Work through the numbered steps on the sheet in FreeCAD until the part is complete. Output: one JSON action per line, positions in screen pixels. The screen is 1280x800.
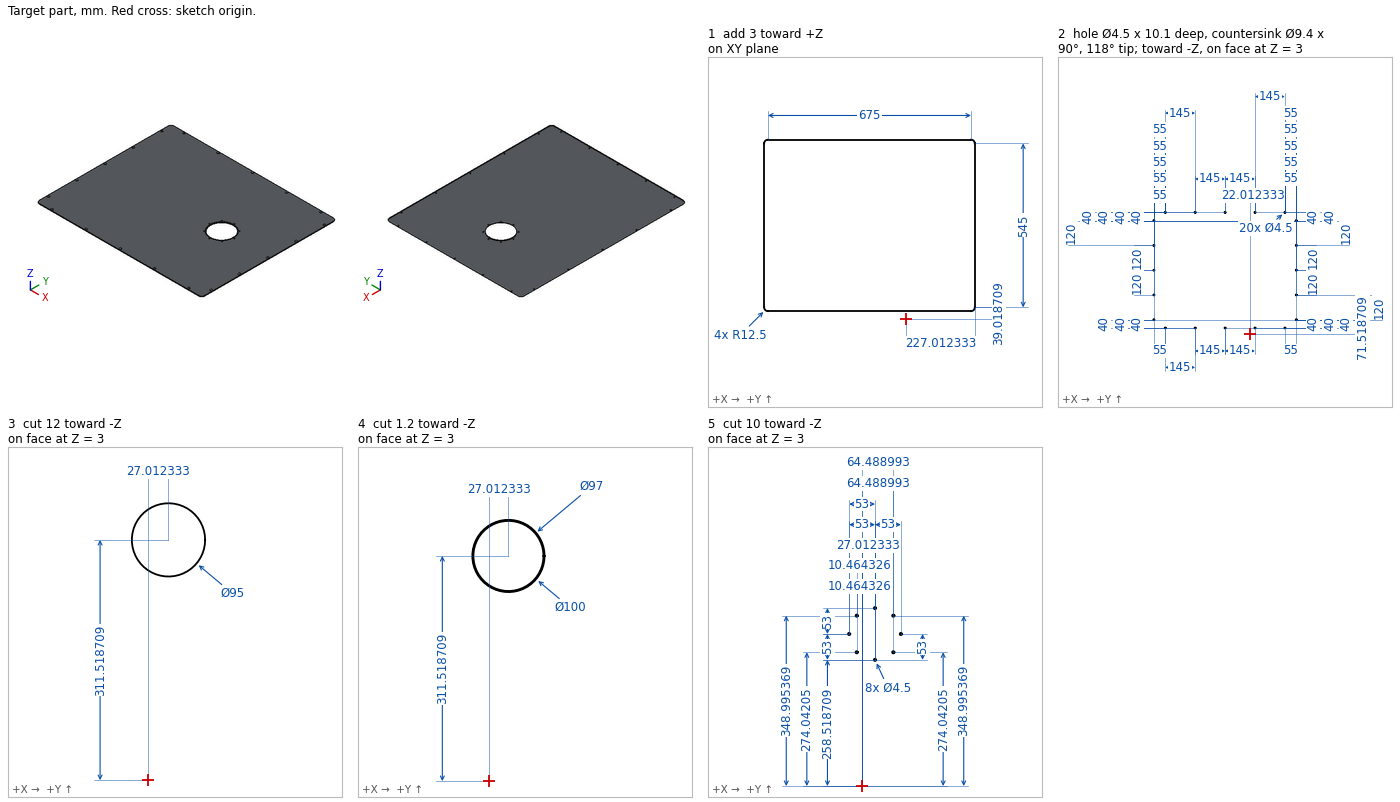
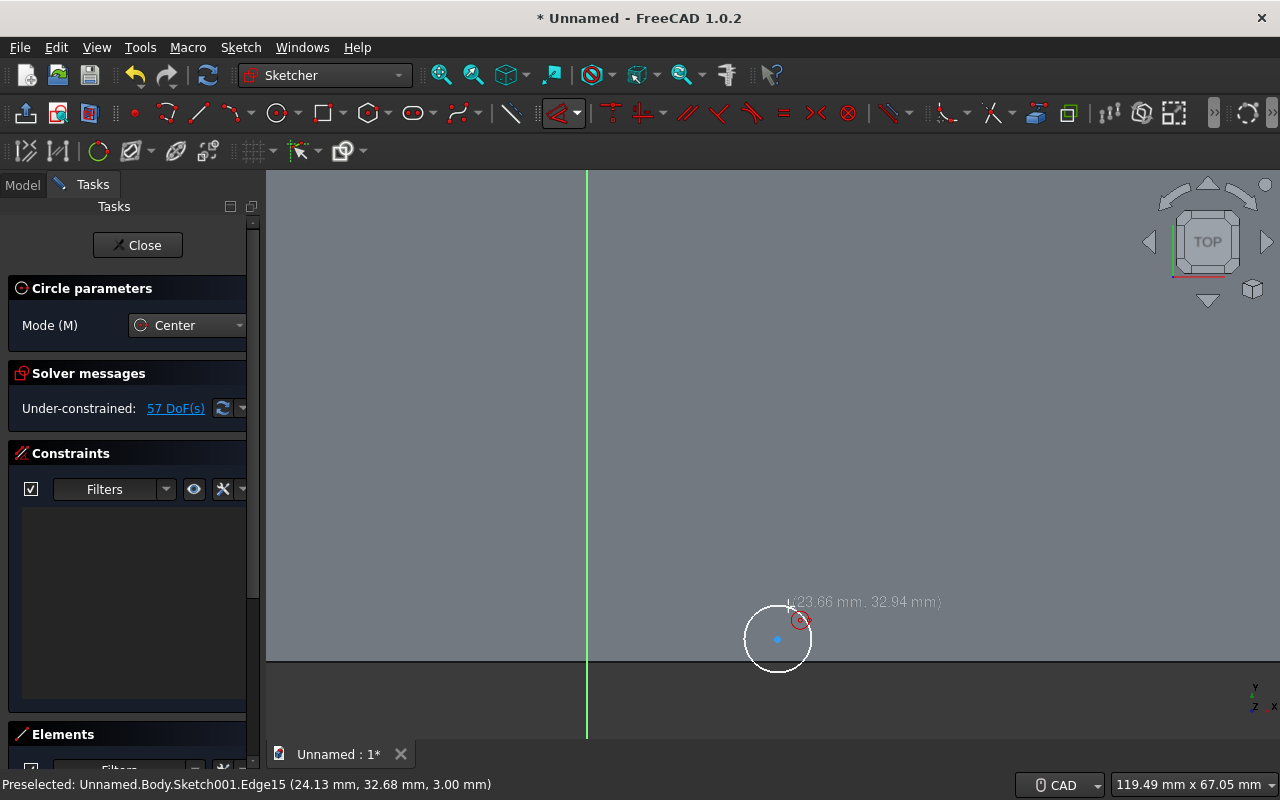
{"action": "scroll", "coordinate": [798, 622], "scroll_direction": "down", "scroll_amount": 13}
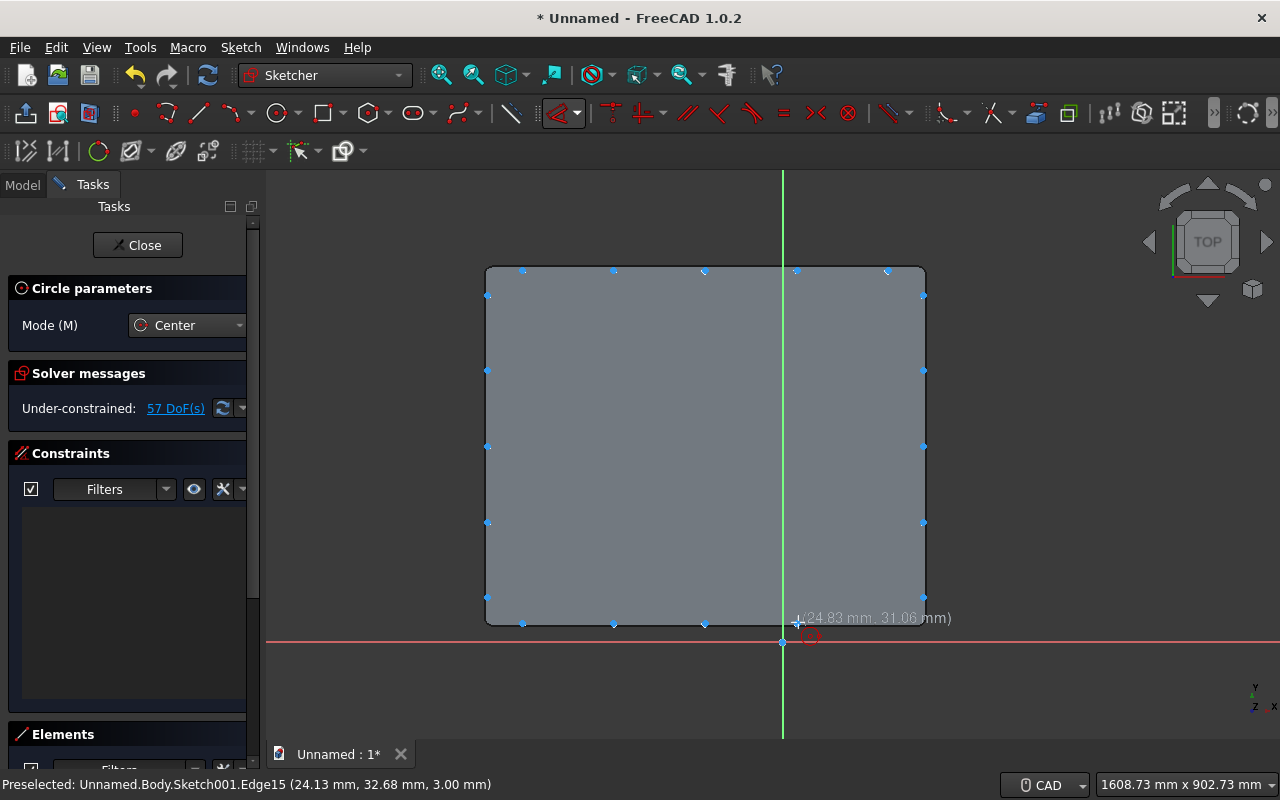
{"action": "scroll", "coordinate": [888, 623], "scroll_direction": "up", "scroll_amount": 14}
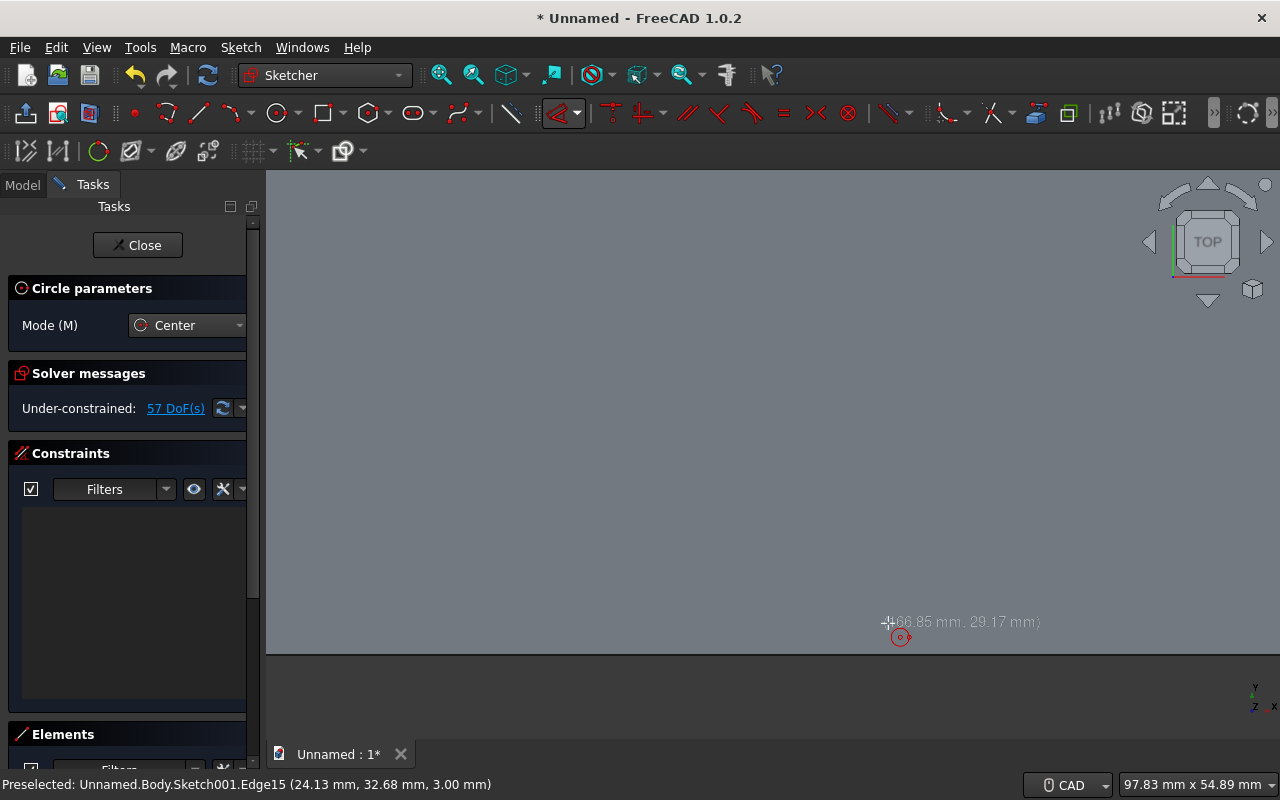
{"action": "scroll", "coordinate": [888, 623], "scroll_direction": "down", "scroll_amount": 14}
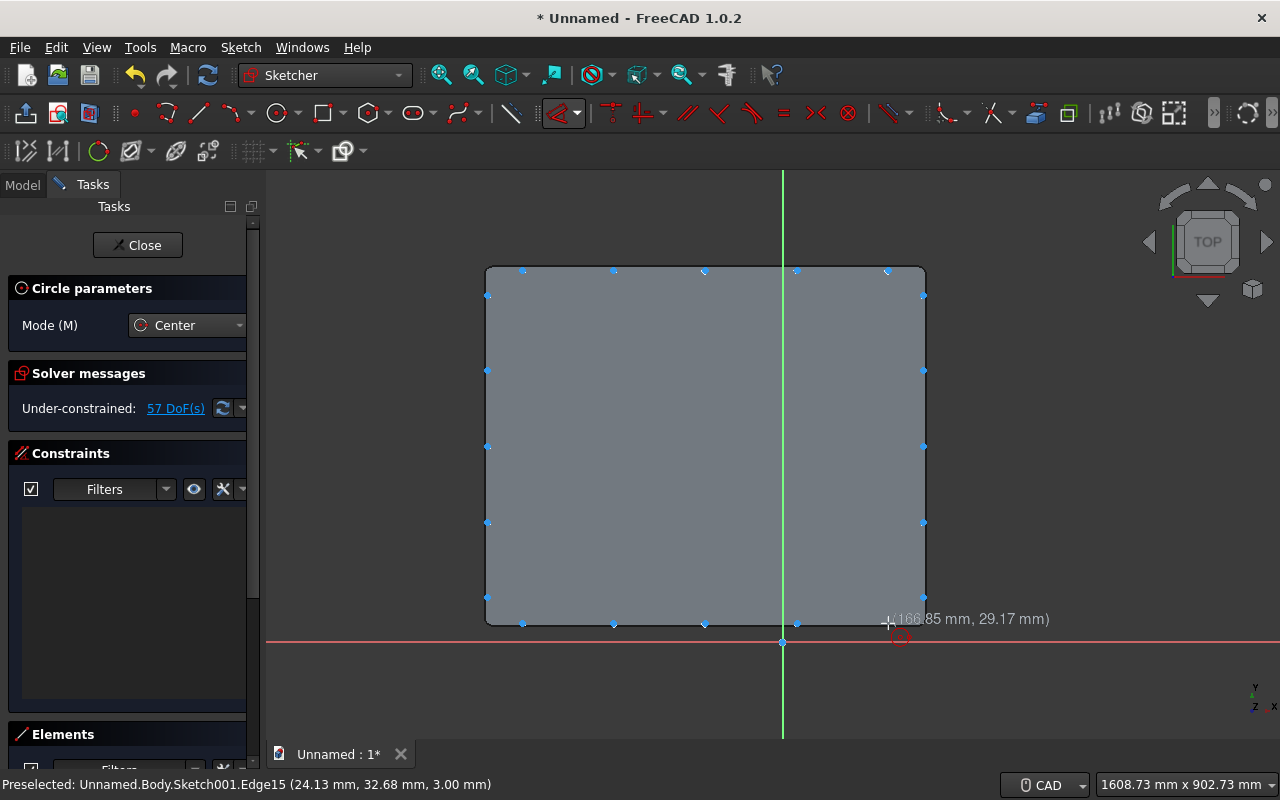
{"action": "left_click", "coordinate": [888, 623]}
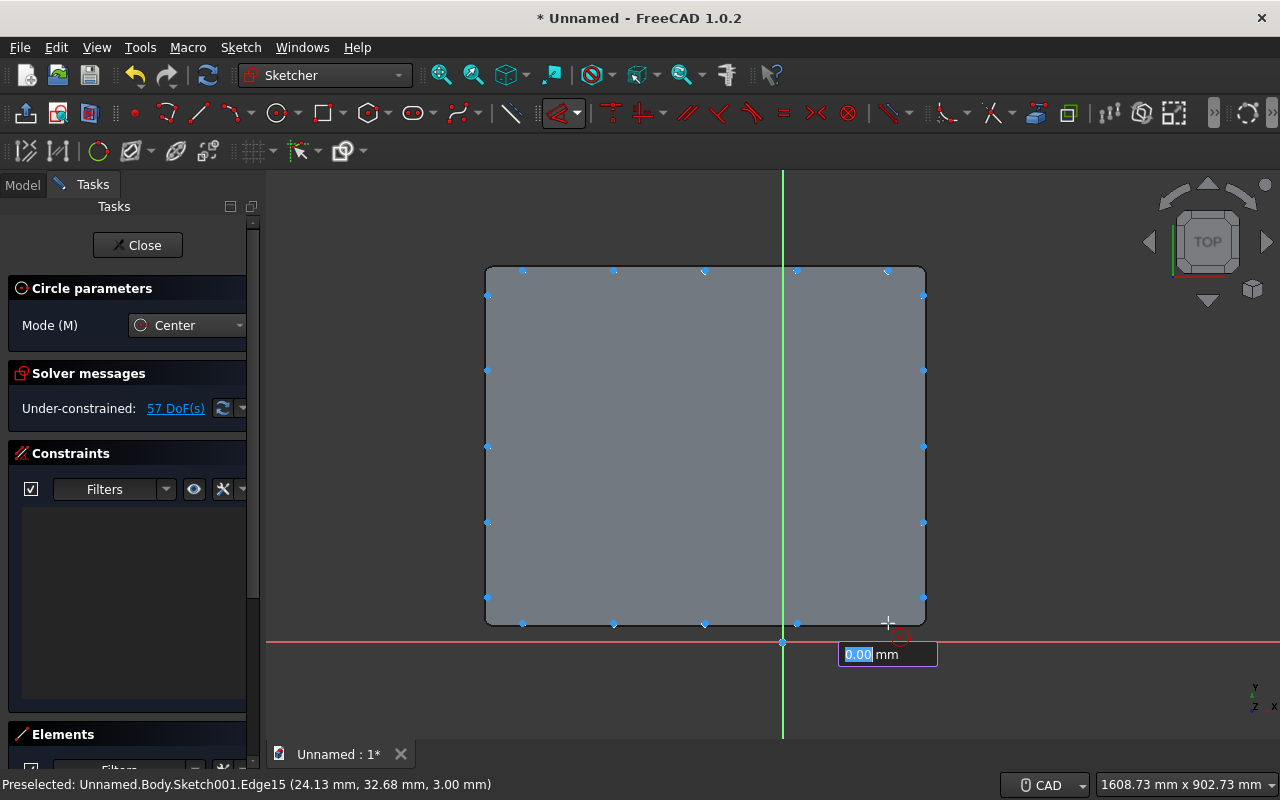
{"action": "scroll", "coordinate": [889, 622], "scroll_direction": "up", "scroll_amount": 13}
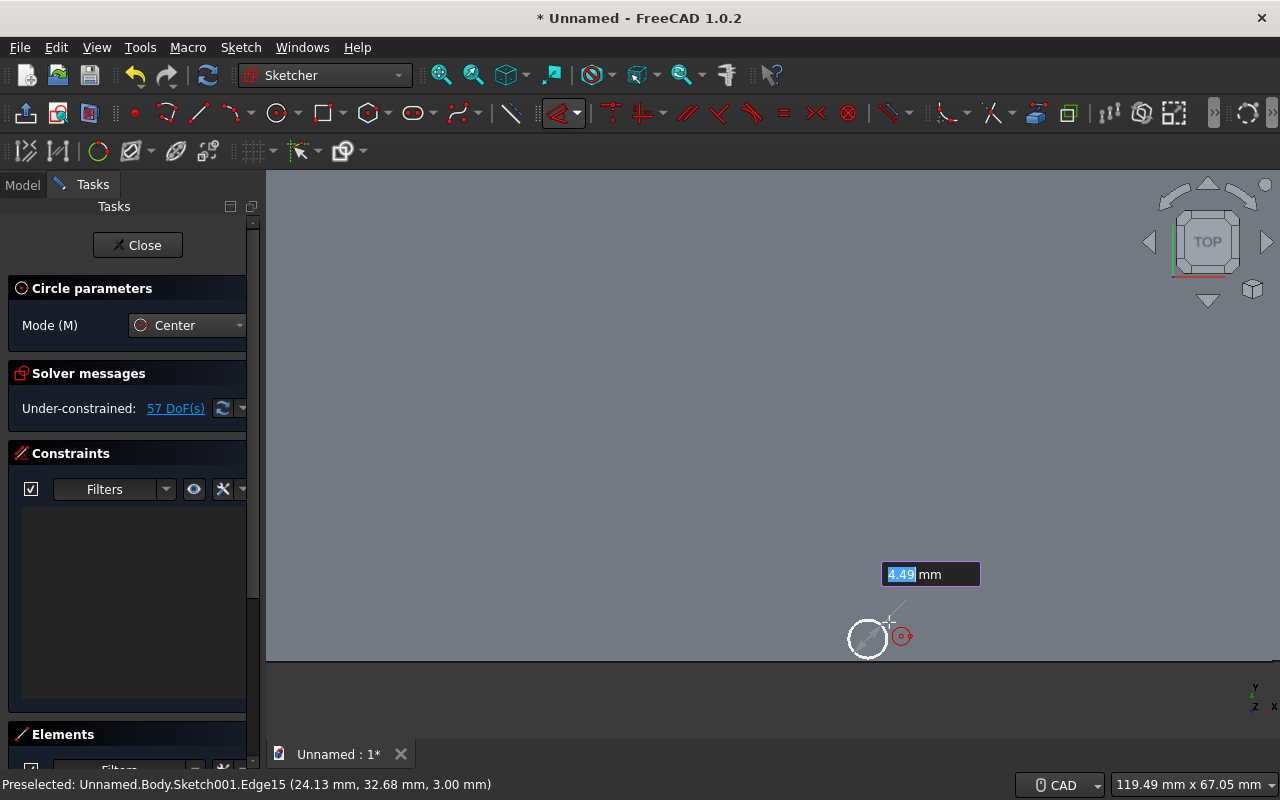
{"action": "left_click", "coordinate": [883, 606]}
{"action": "key", "text": "Escape"}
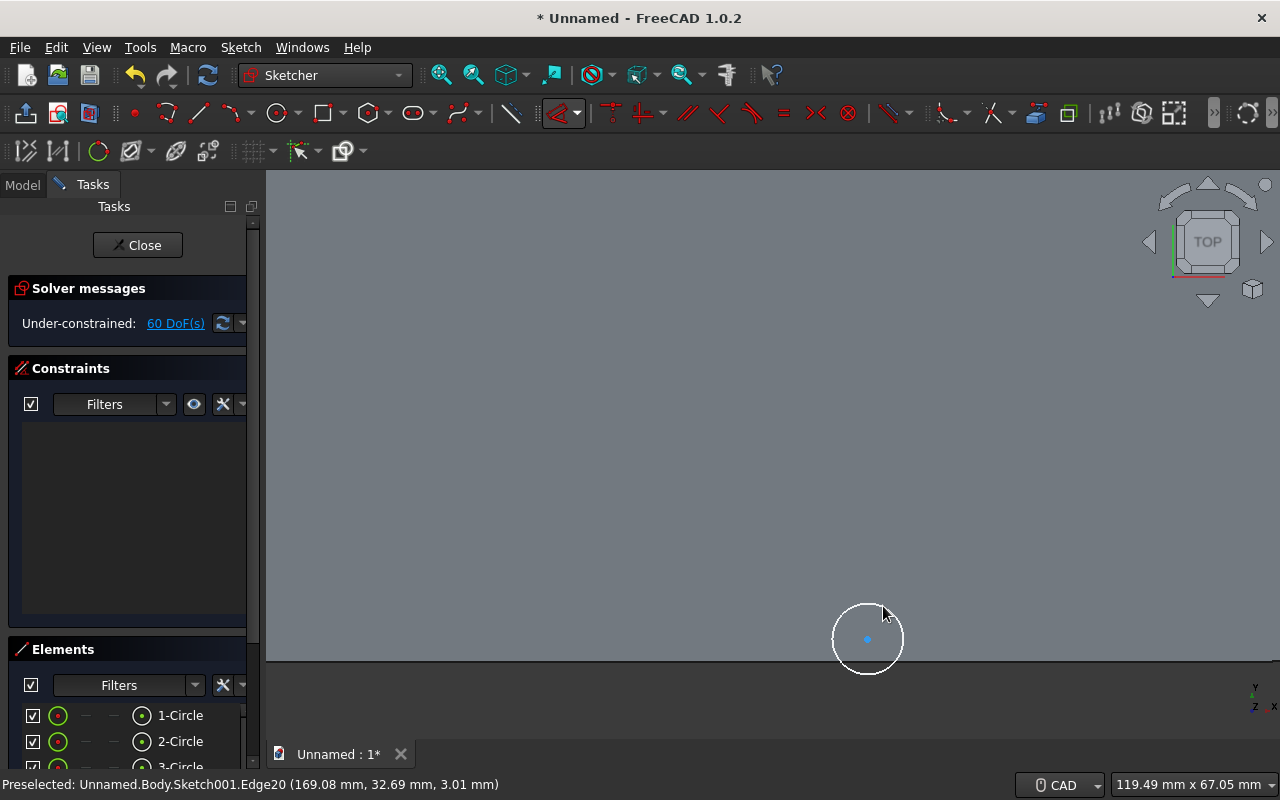
{"action": "scroll", "coordinate": [889, 622], "scroll_direction": "down", "scroll_amount": 13}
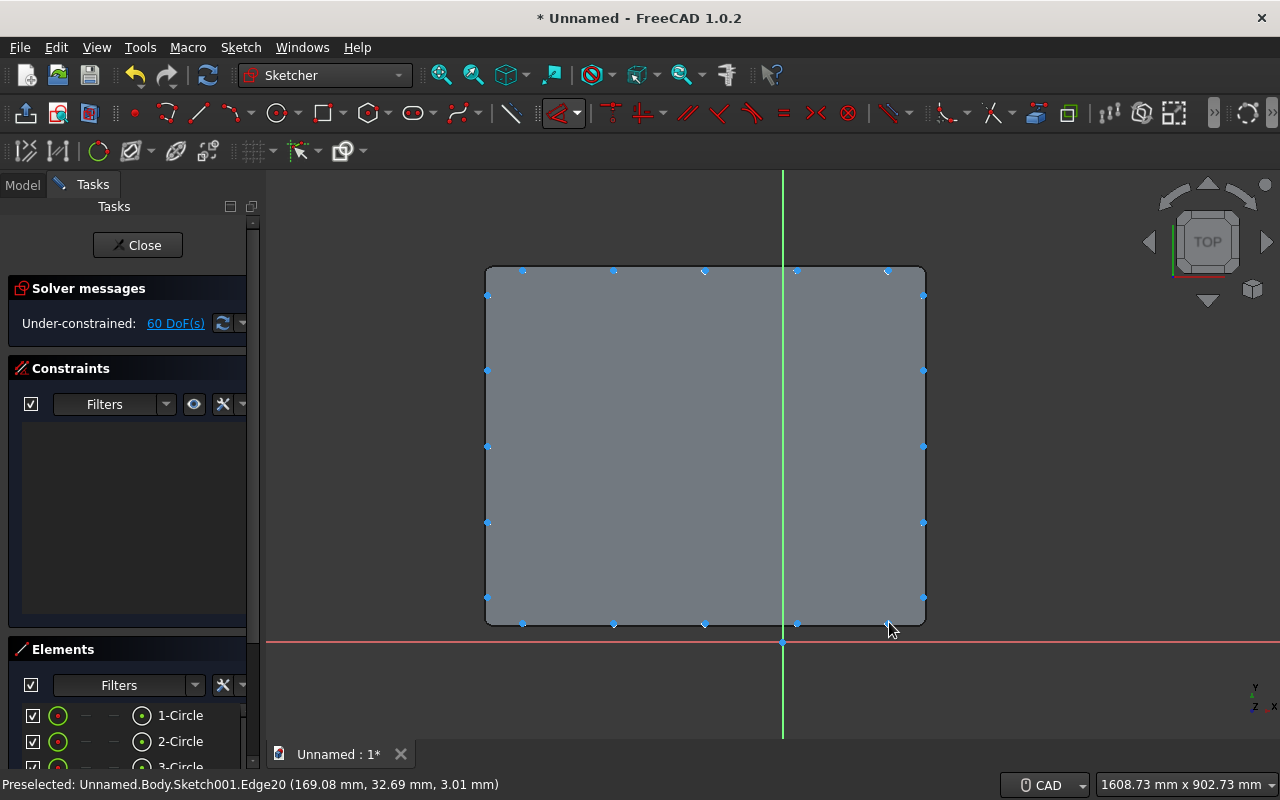
{"action": "scroll", "coordinate": [924, 597], "scroll_direction": "up", "scroll_amount": 11}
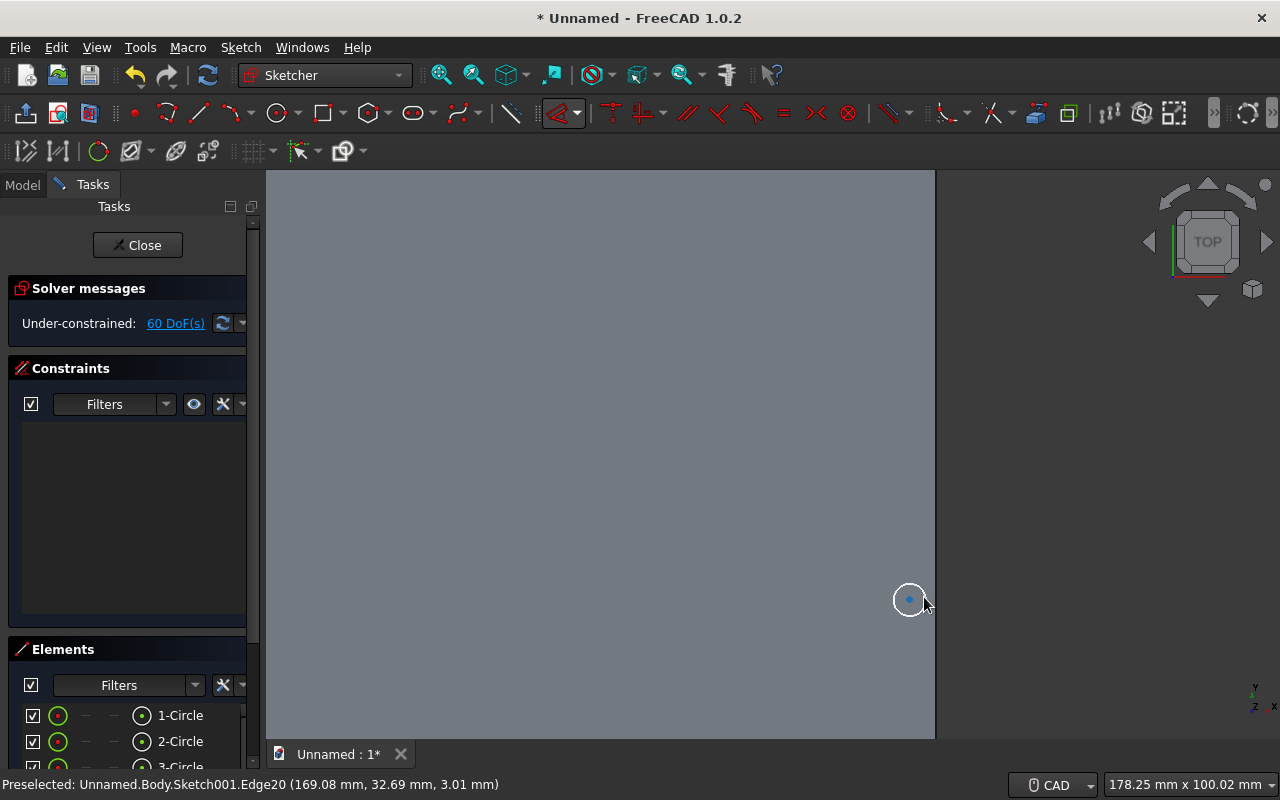
{"action": "left_click", "coordinate": [921, 589]}